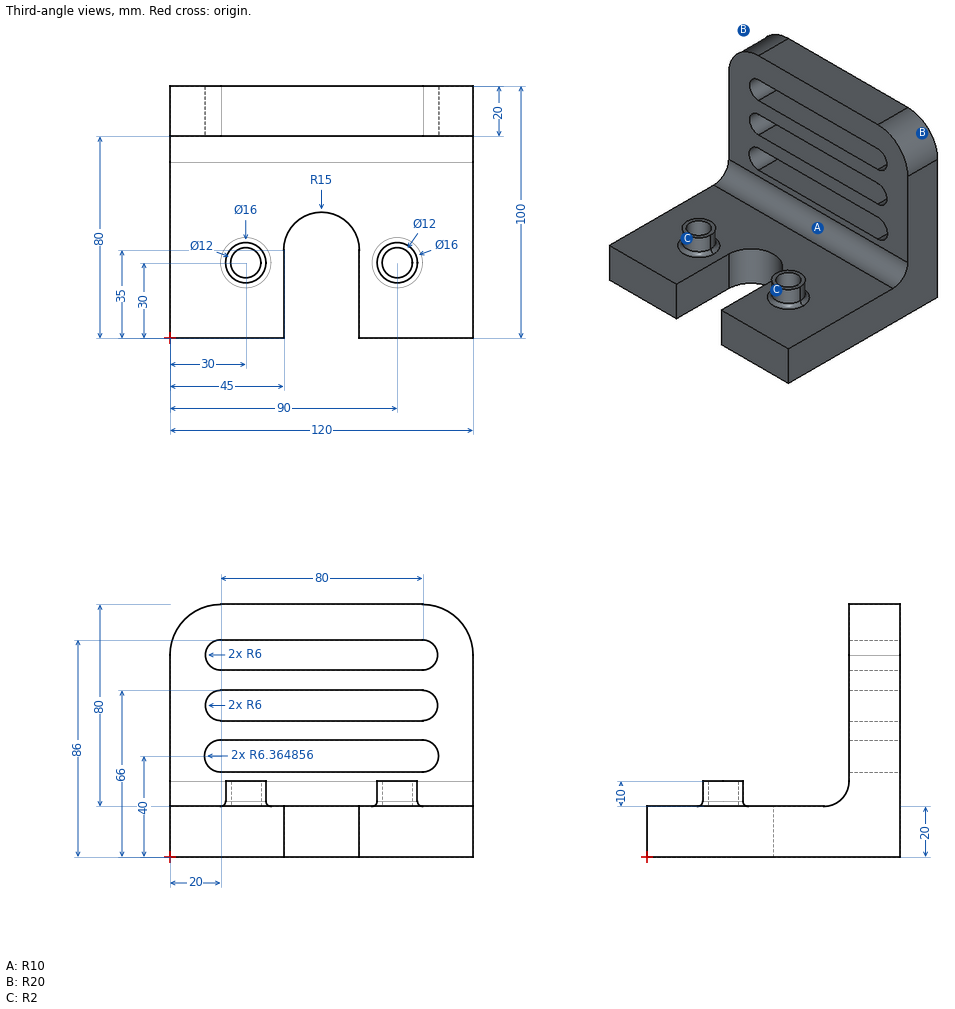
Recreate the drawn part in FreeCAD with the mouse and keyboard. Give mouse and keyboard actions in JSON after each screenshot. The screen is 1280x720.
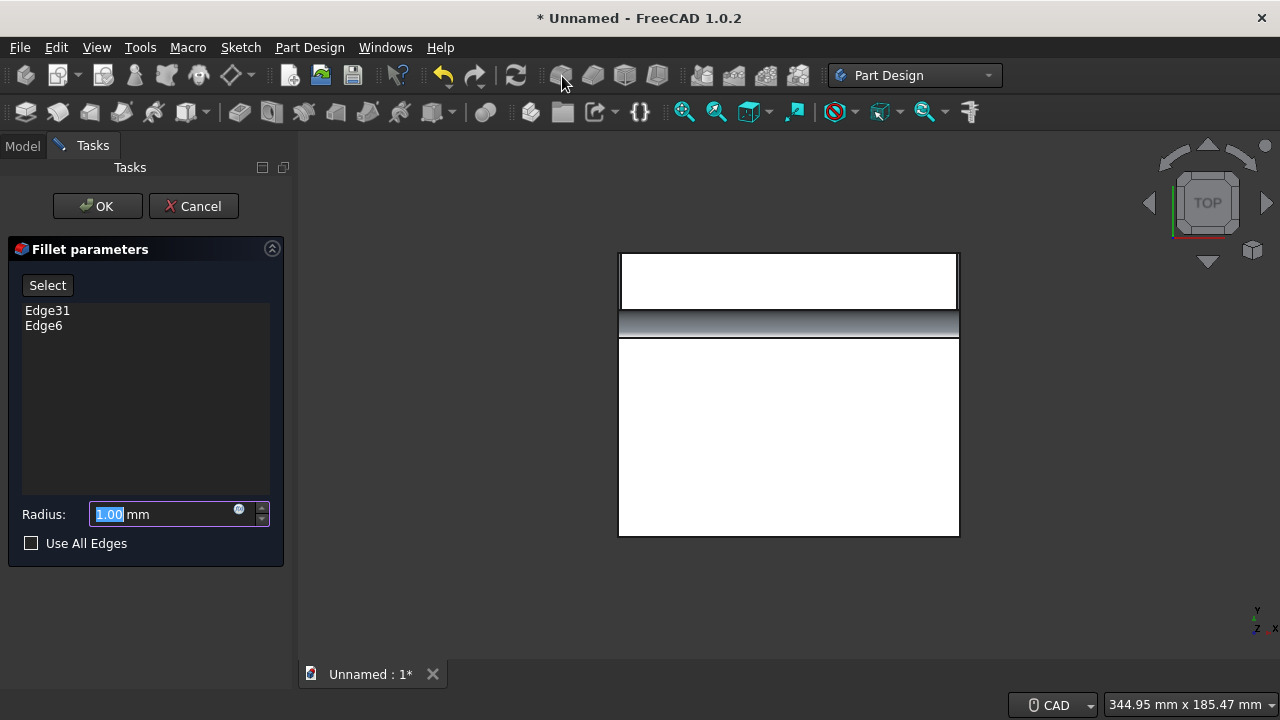
{"action": "type", "text": "20"}
{"action": "key", "text": "Tab"}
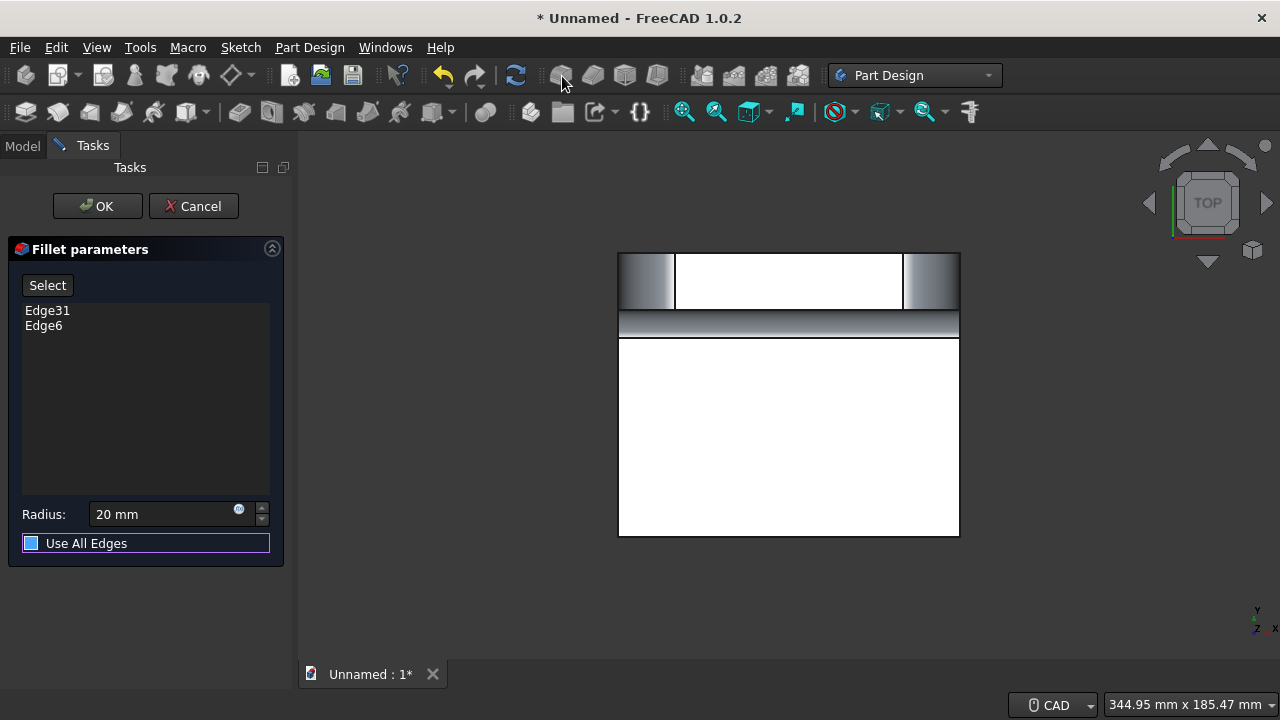
{"action": "left_click", "coordinate": [98, 206]}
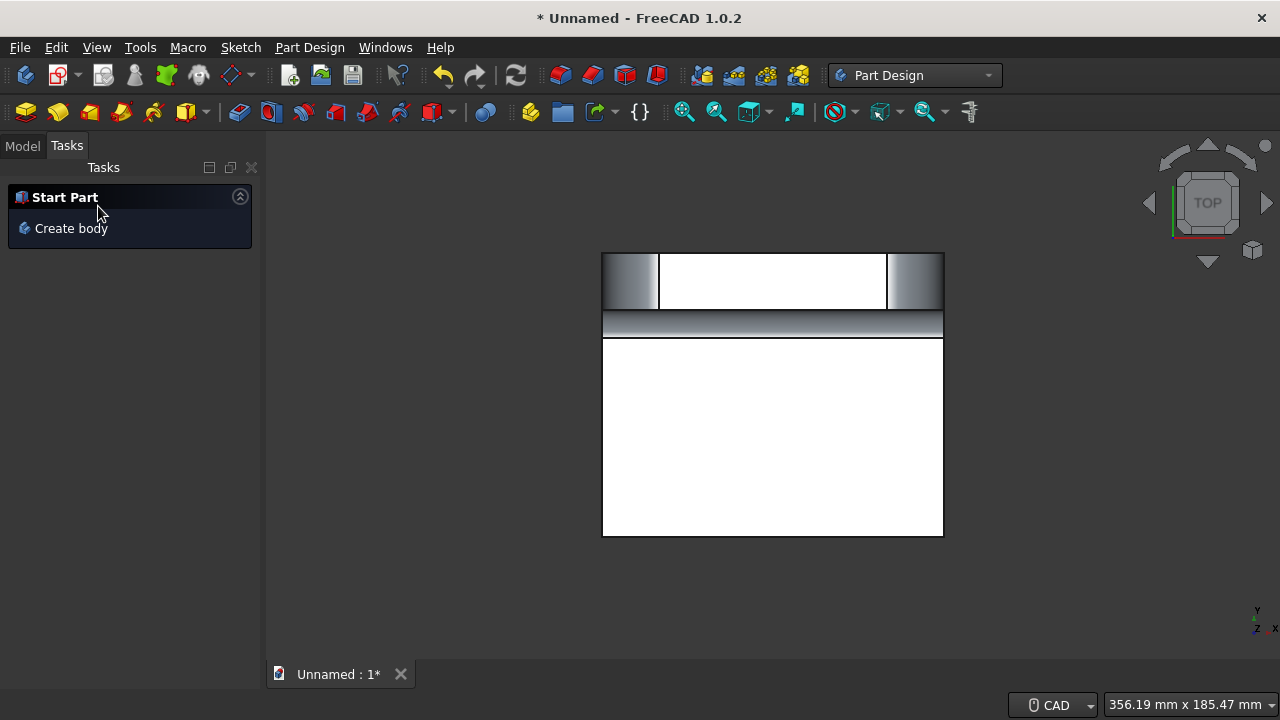
{"action": "left_click", "coordinate": [822, 437]}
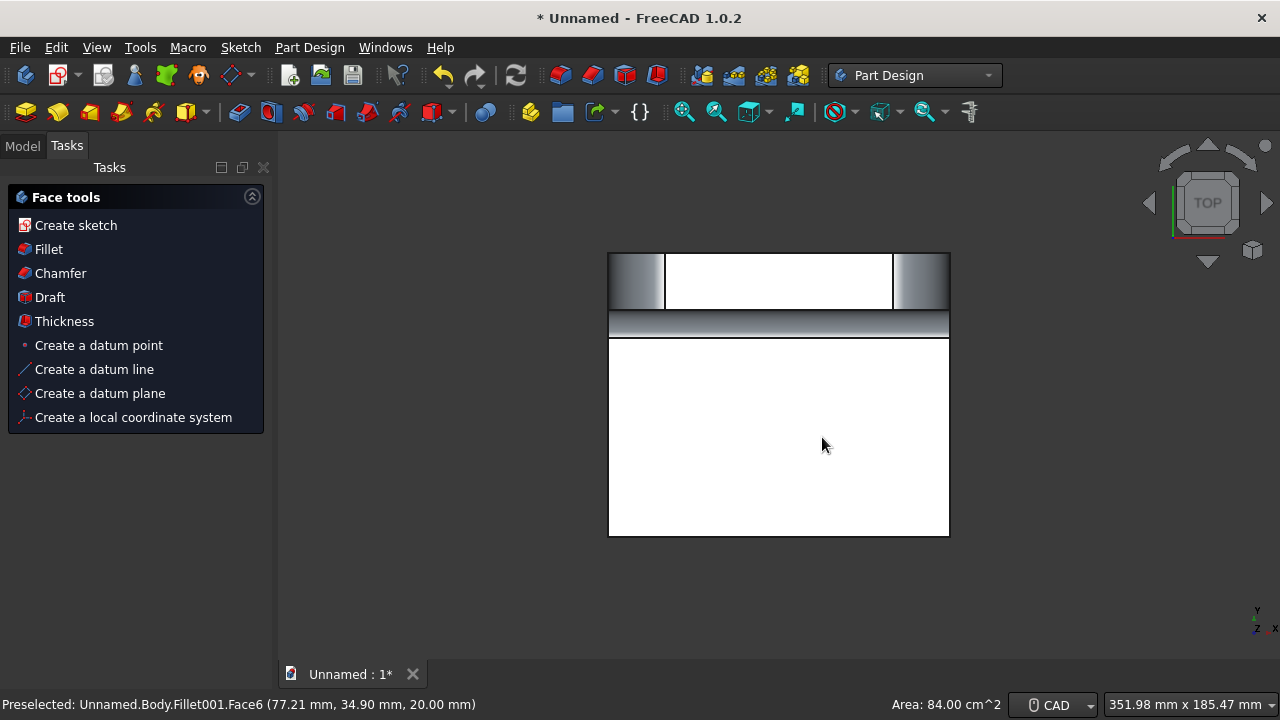
{"action": "left_click", "coordinate": [58, 76]}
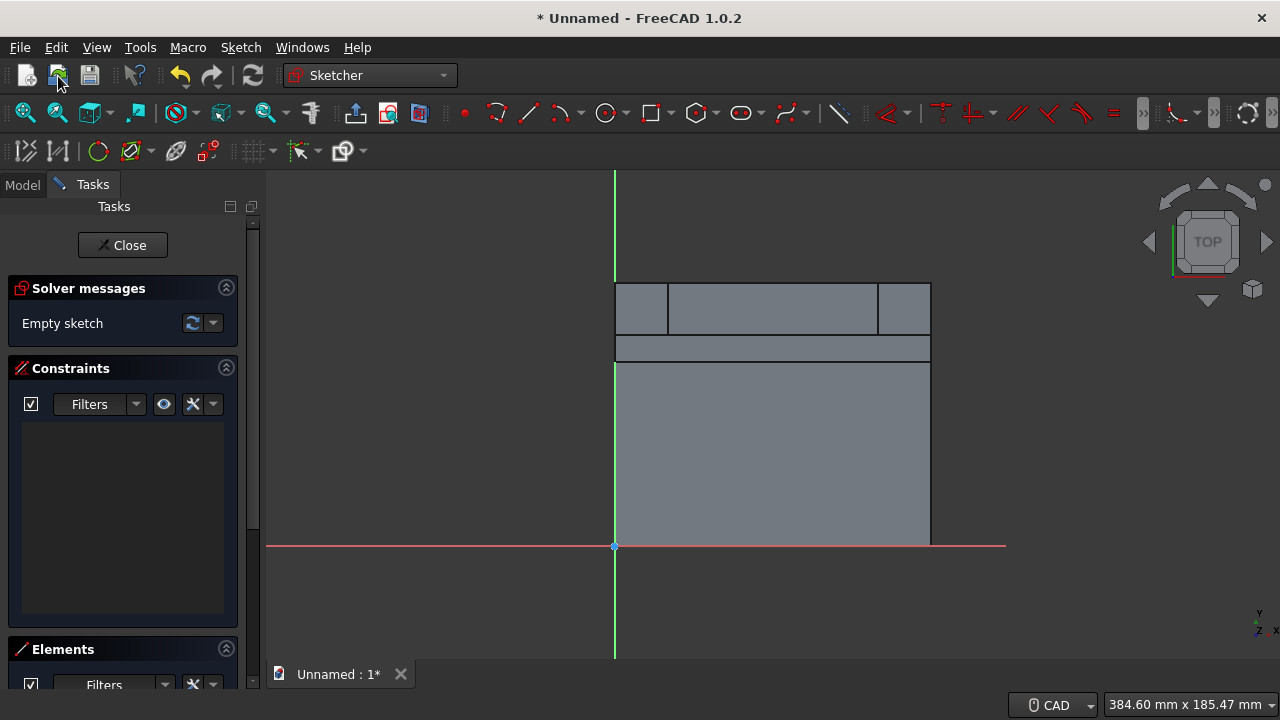
{"action": "left_click", "coordinate": [420, 114]}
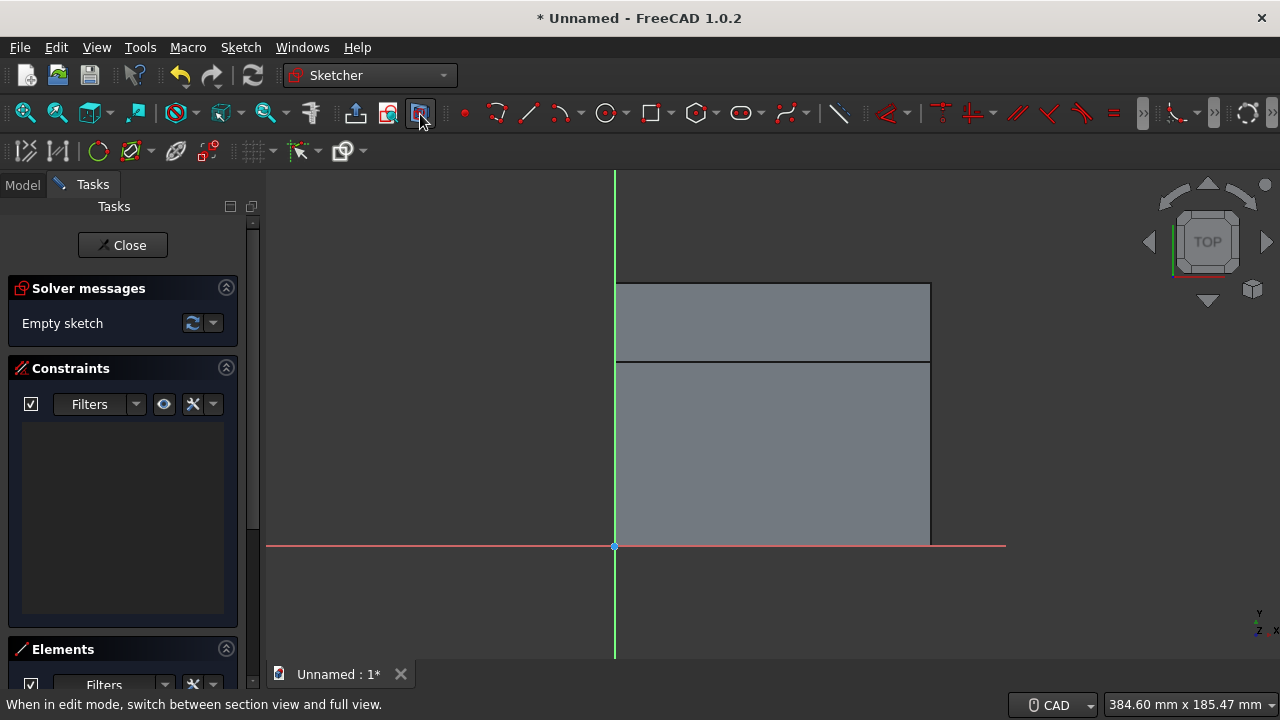
{"action": "scroll", "coordinate": [721, 534], "scroll_direction": "up", "scroll_amount": 4}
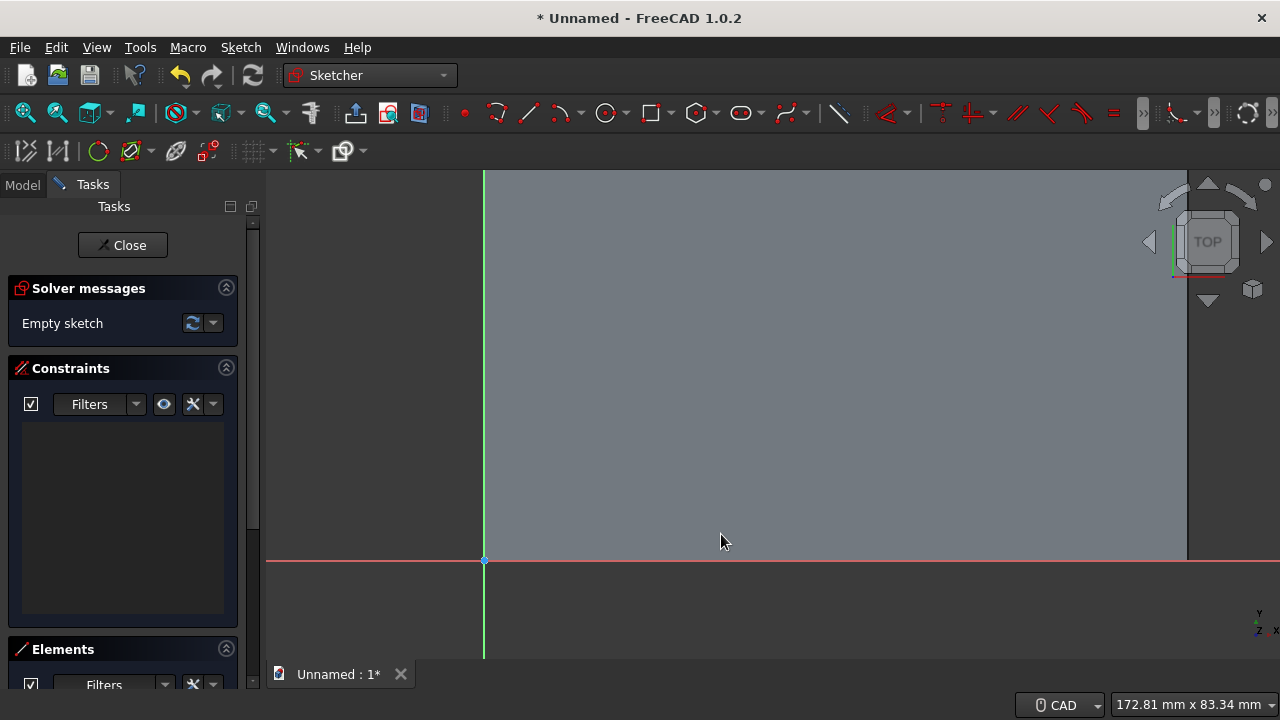
{"action": "left_click", "coordinate": [498, 114]}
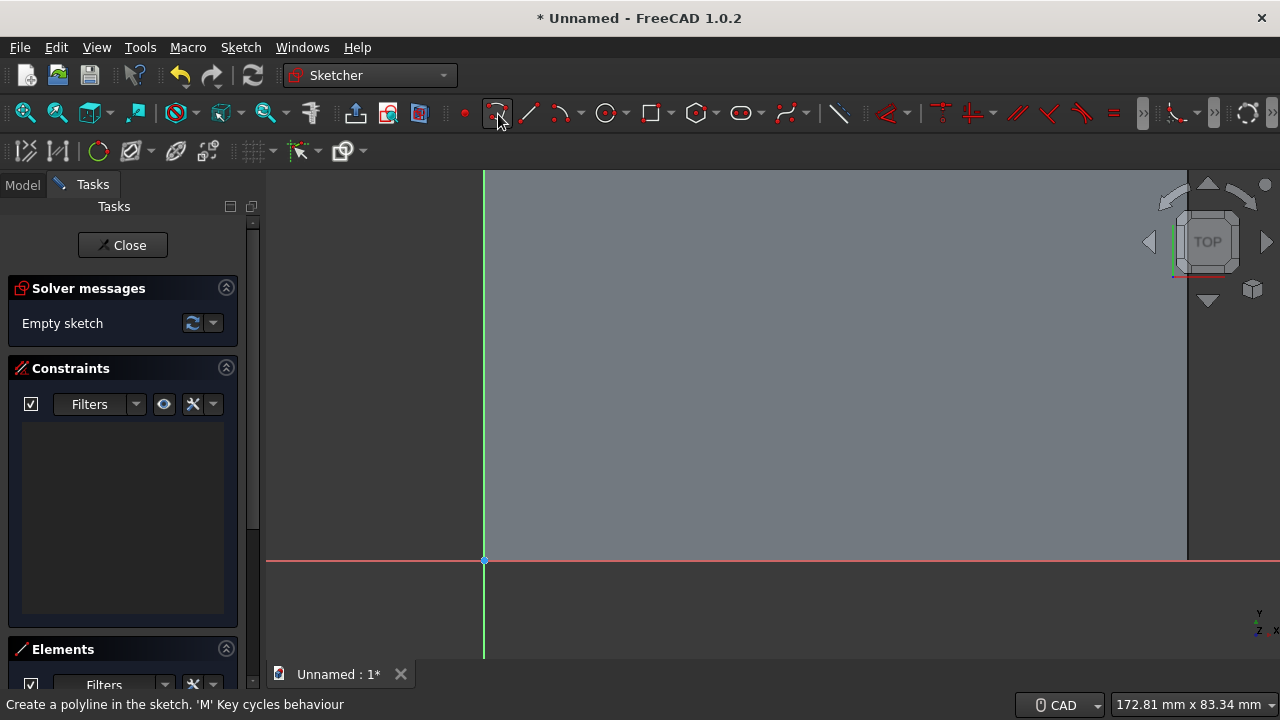
{"action": "left_click", "coordinate": [748, 355]}
{"action": "left_click", "coordinate": [748, 561]}
{"action": "left_click", "coordinate": [924, 552]}
{"action": "left_click", "coordinate": [924, 355]}
{"action": "right_click", "coordinate": [924, 355]}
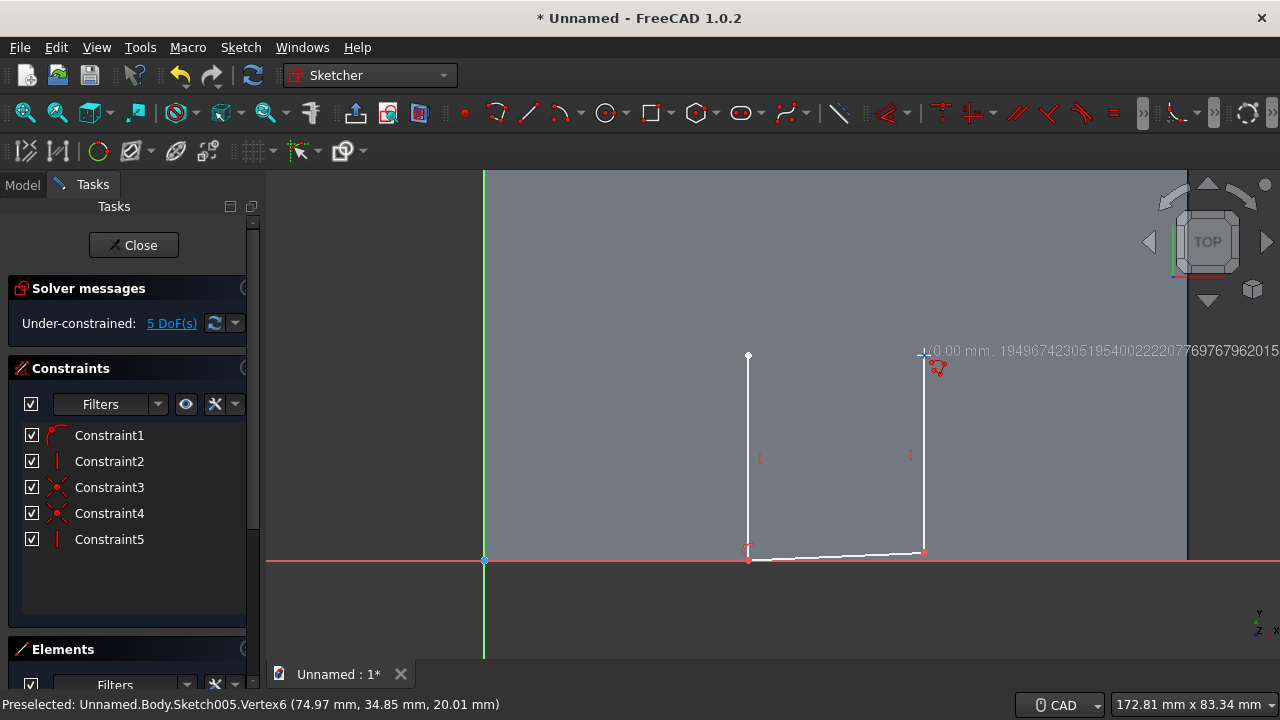
{"action": "key", "text": "g 3 a"}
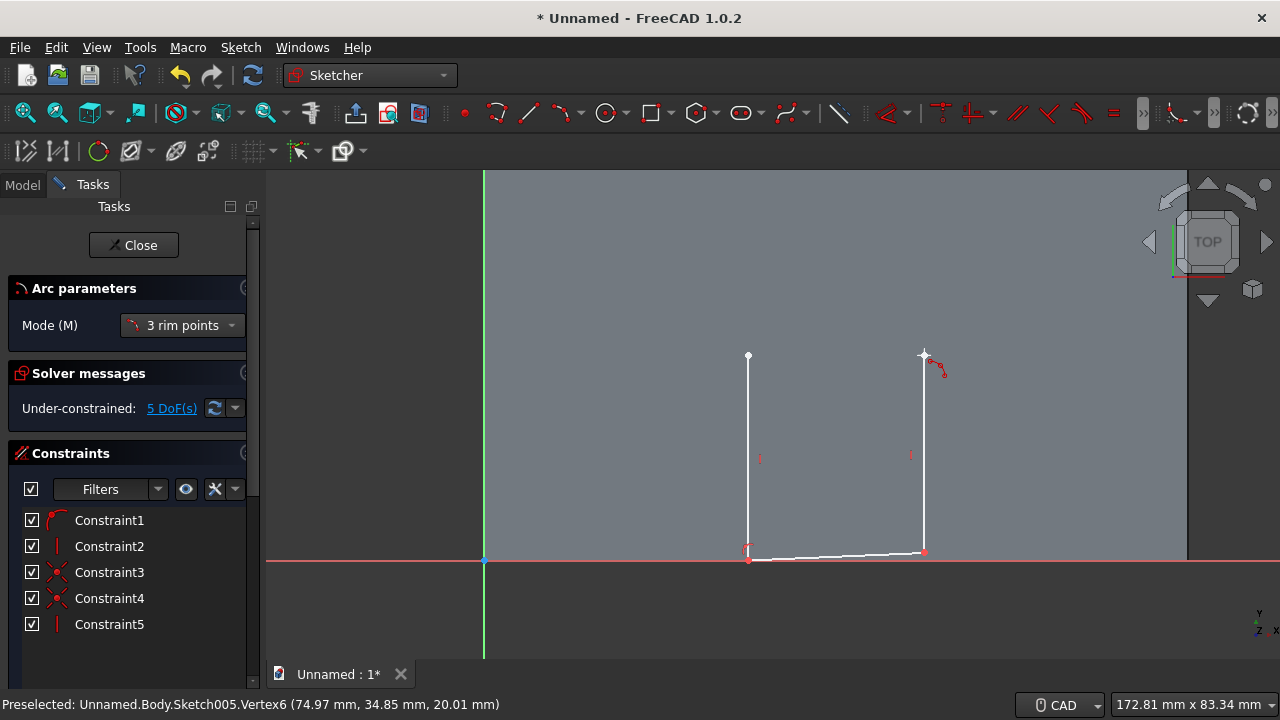
{"action": "left_click", "coordinate": [924, 356]}
{"action": "left_click", "coordinate": [748, 356]}
{"action": "left_click", "coordinate": [836, 267]}
{"action": "key", "text": "Escape"}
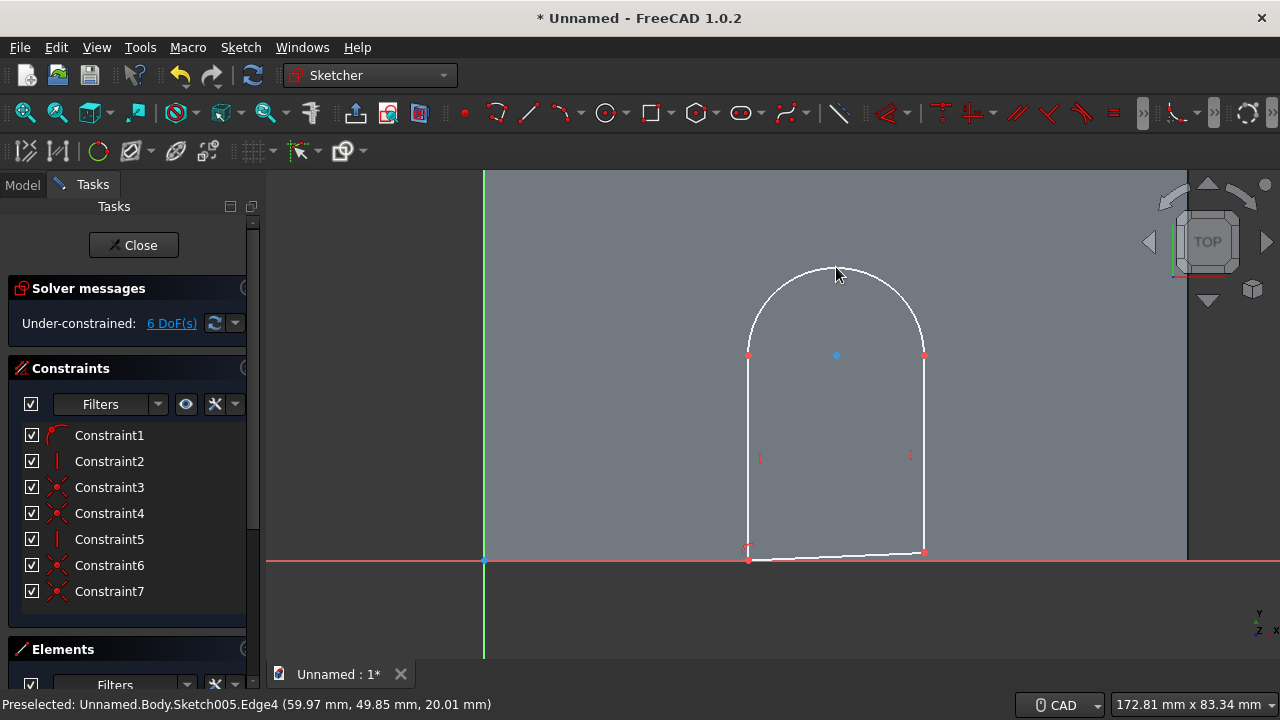
{"action": "left_click", "coordinate": [748, 417]}